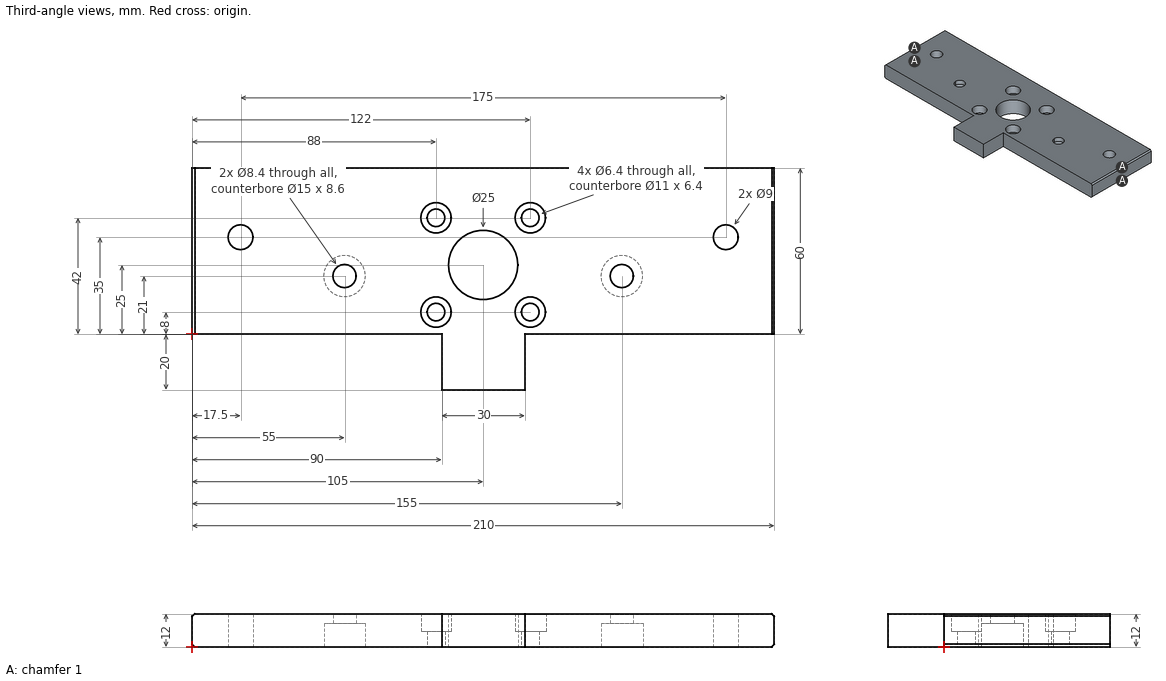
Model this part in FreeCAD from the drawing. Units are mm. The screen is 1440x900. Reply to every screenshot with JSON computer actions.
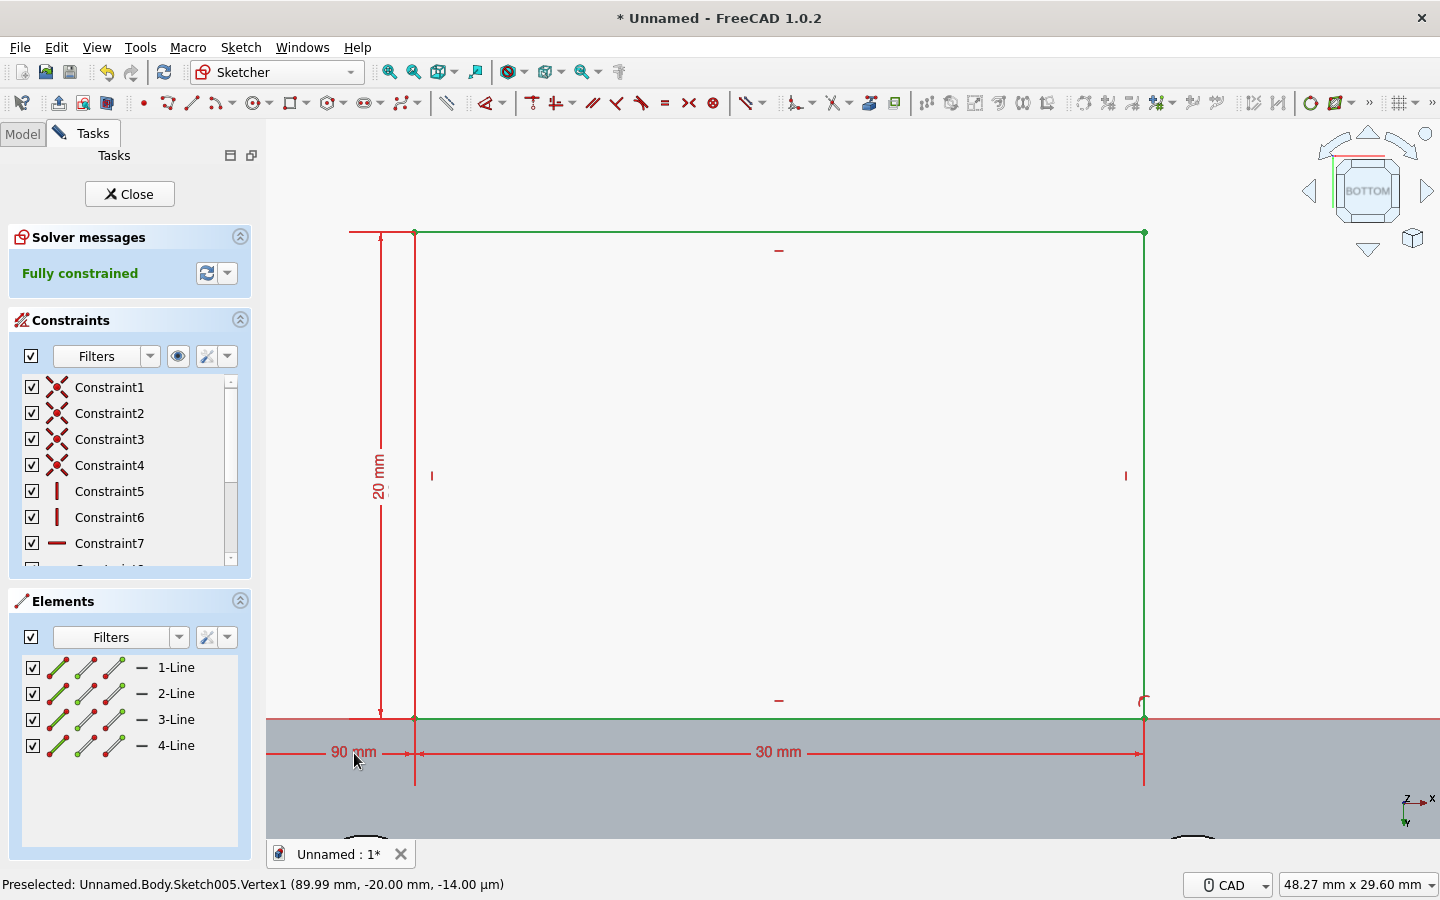
{"action": "left_click", "coordinate": [130, 194]}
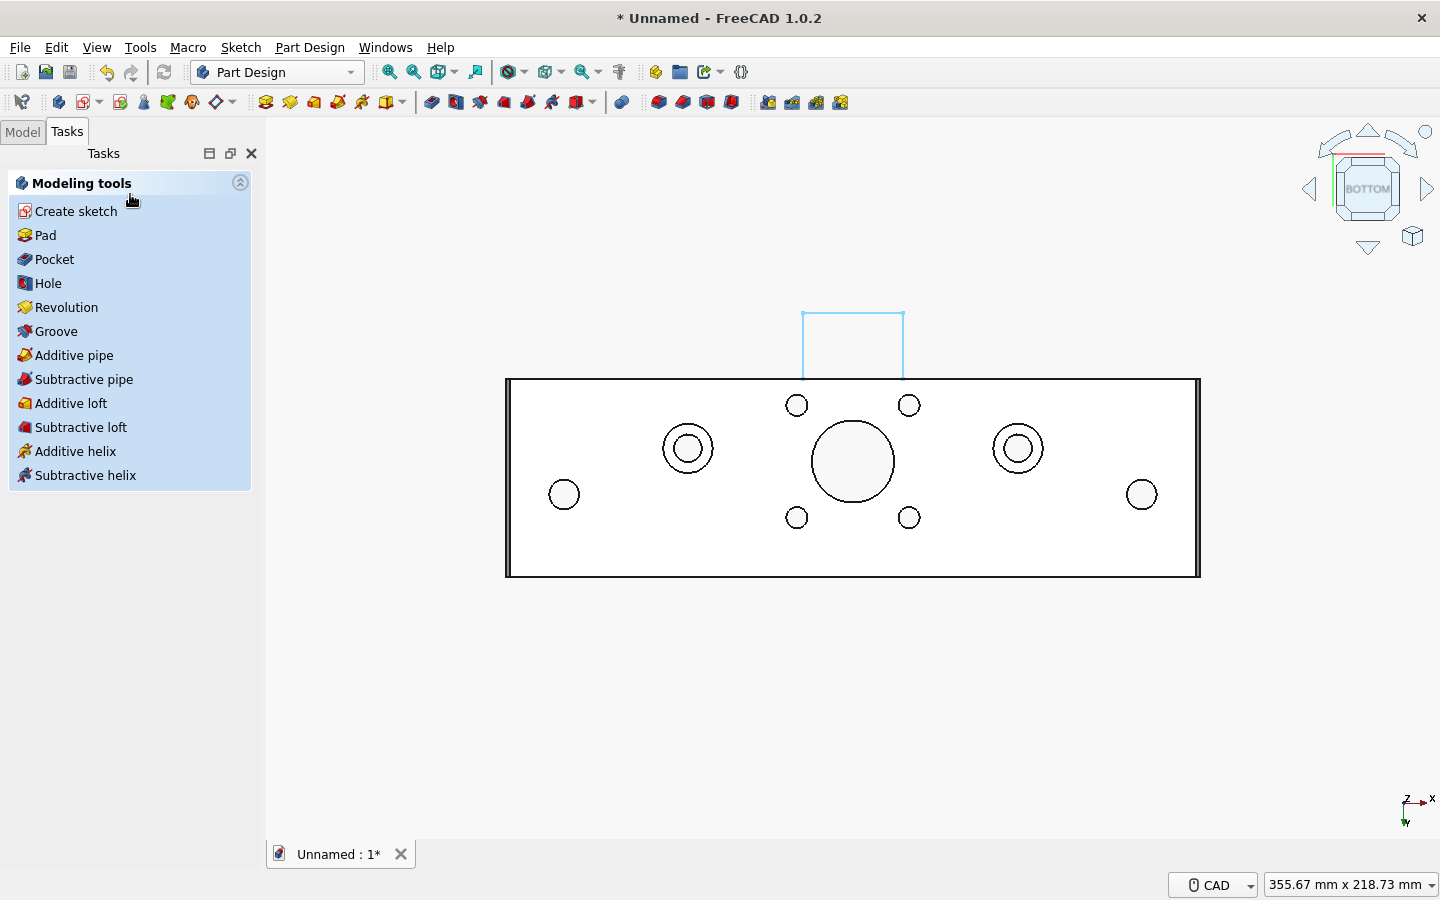
{"action": "left_click", "coordinate": [266, 102]}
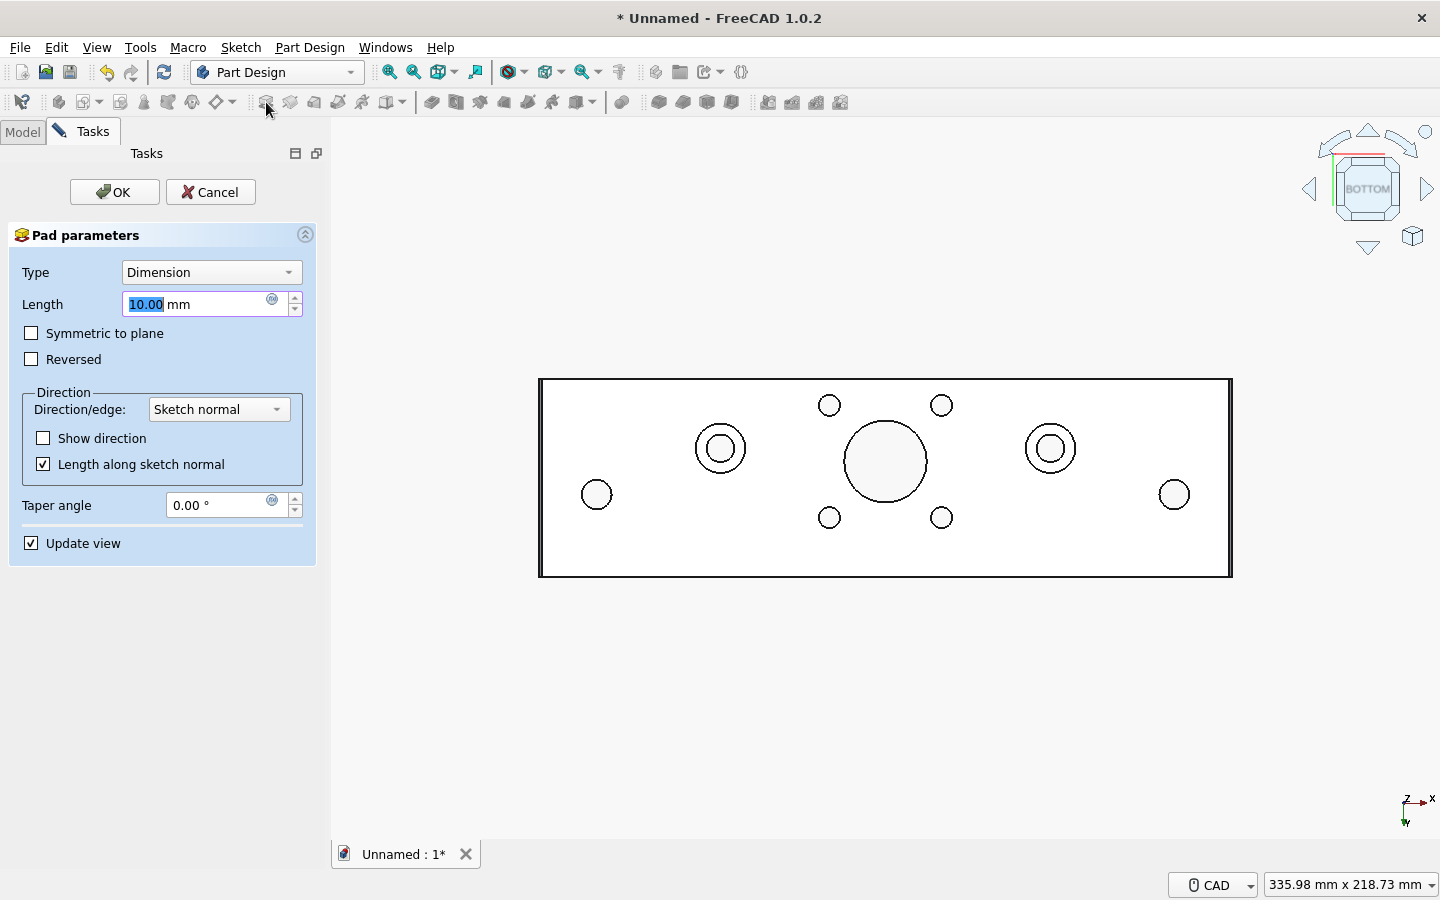
{"action": "type", "text": "12"}
{"action": "key", "text": "Tab"}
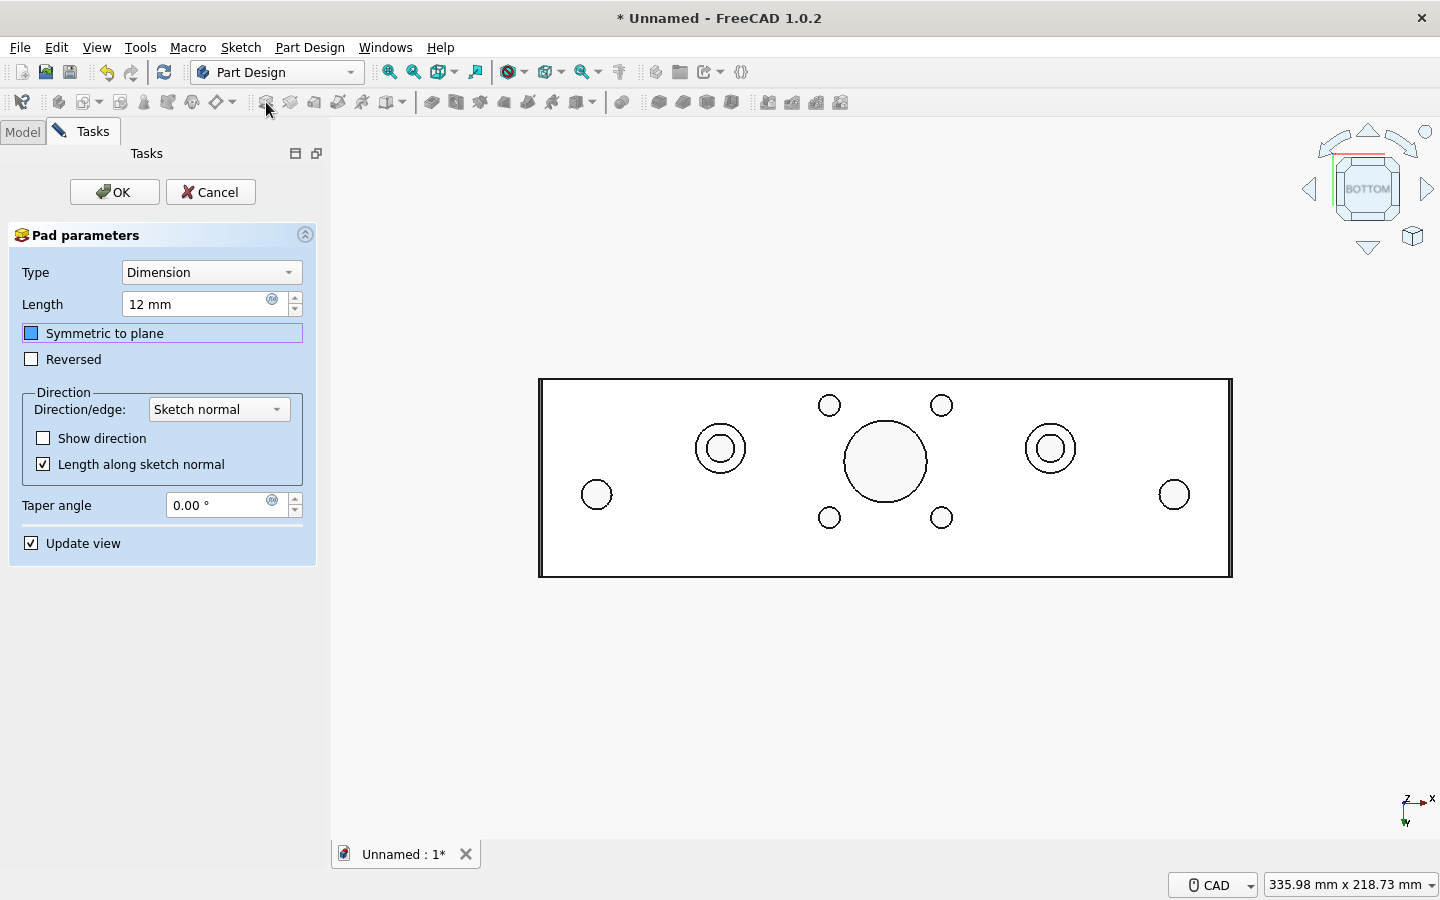
{"action": "left_click", "coordinate": [30, 359]}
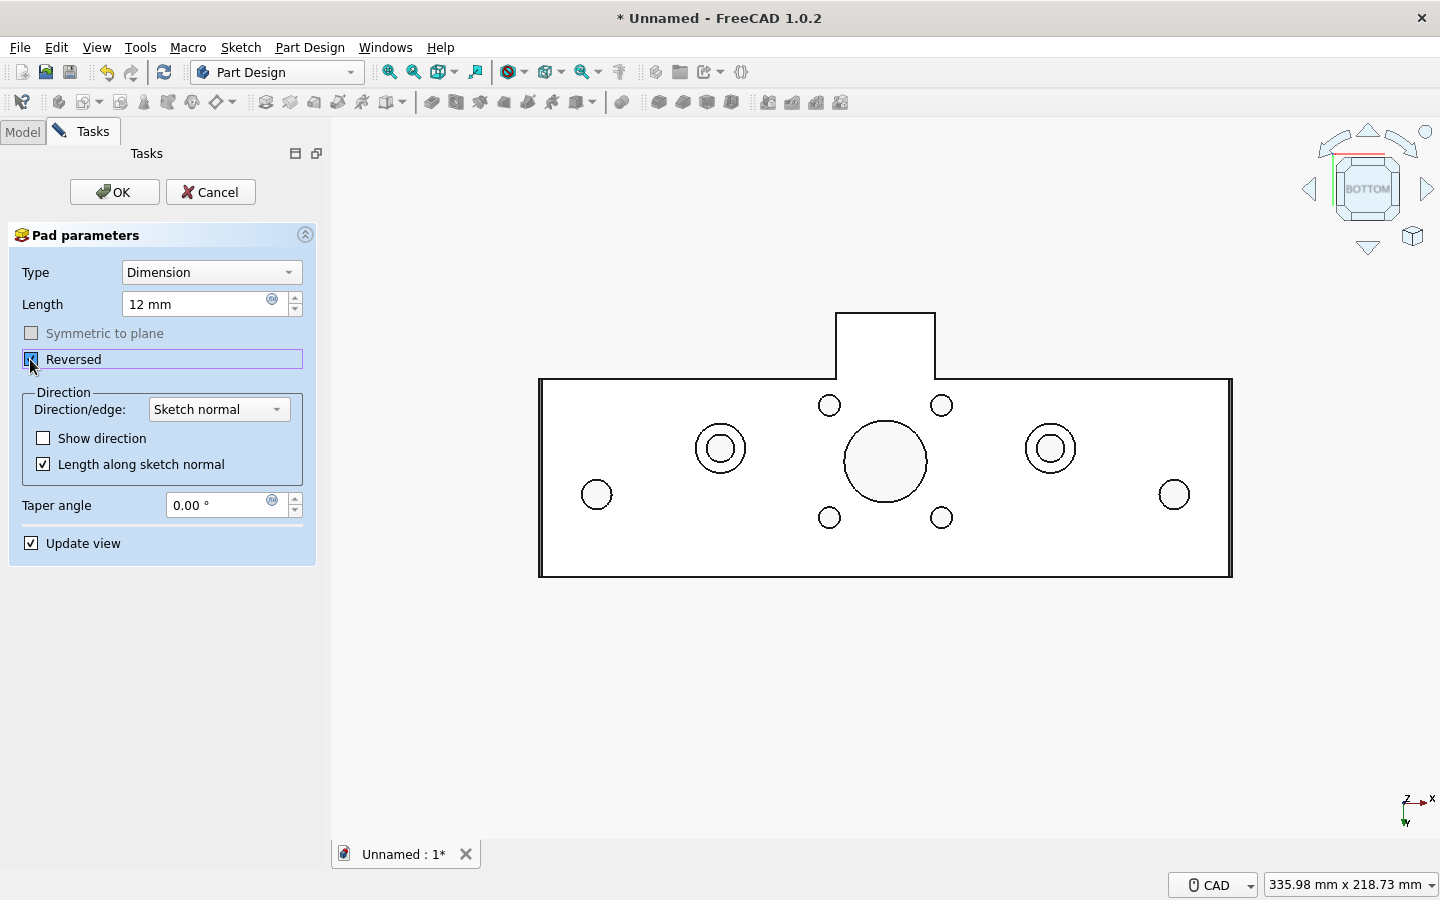
{"action": "left_click", "coordinate": [115, 192]}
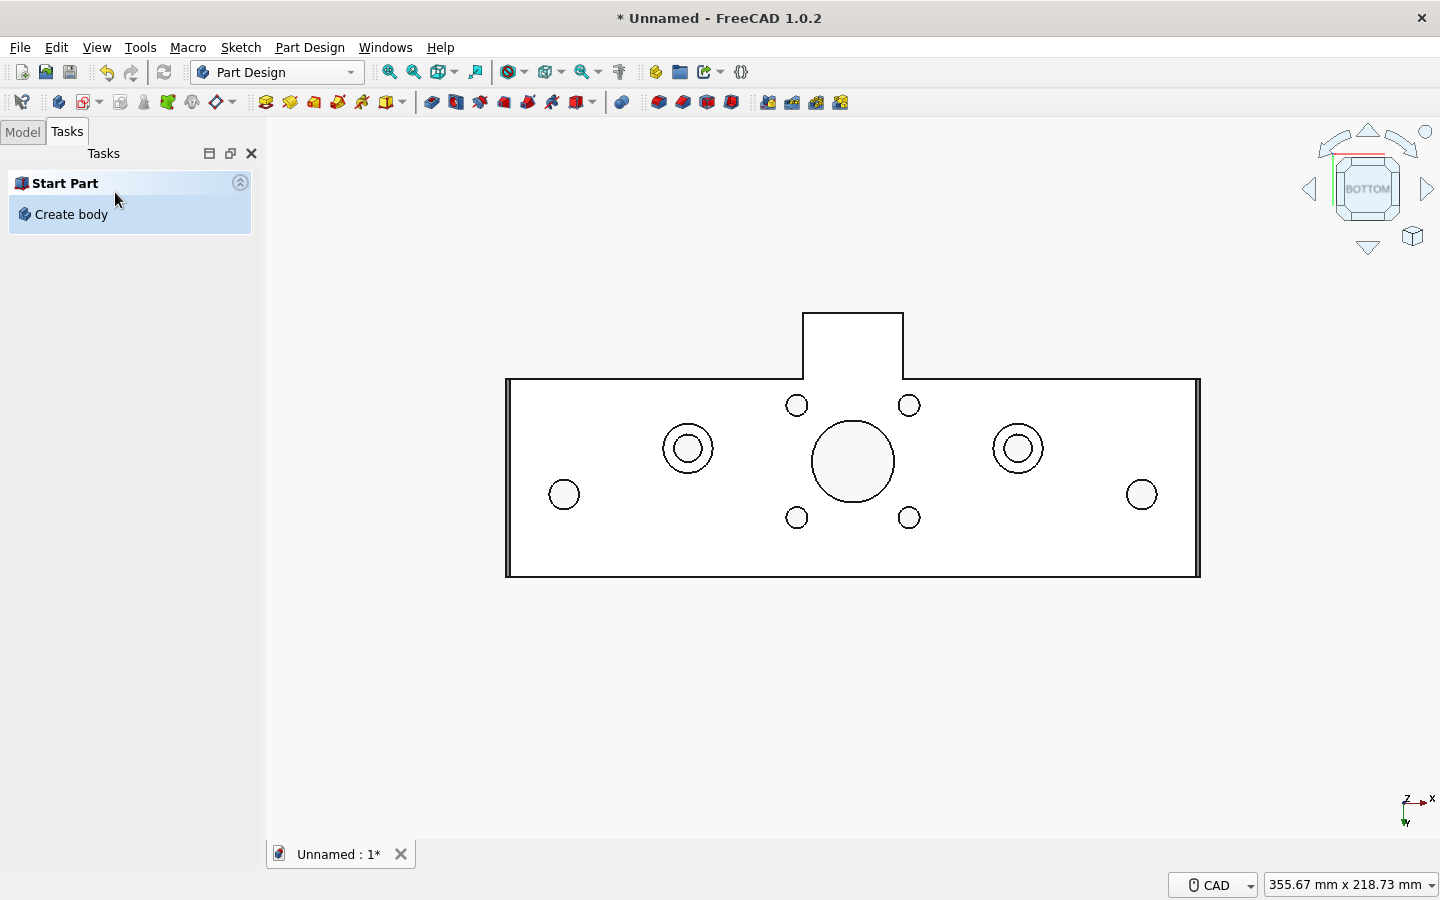
{"action": "key", "text": "0"}